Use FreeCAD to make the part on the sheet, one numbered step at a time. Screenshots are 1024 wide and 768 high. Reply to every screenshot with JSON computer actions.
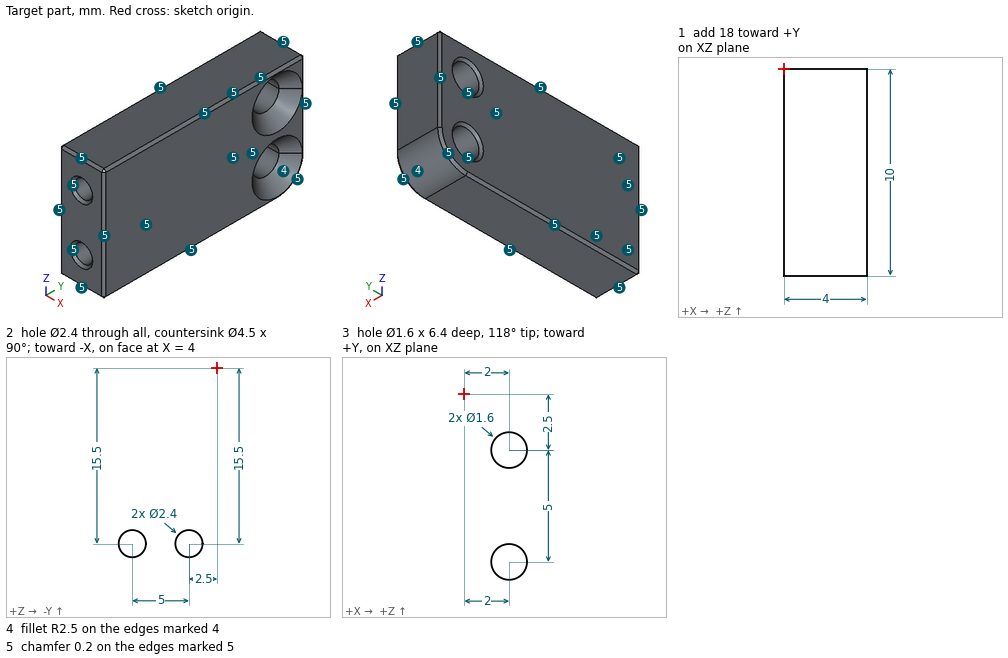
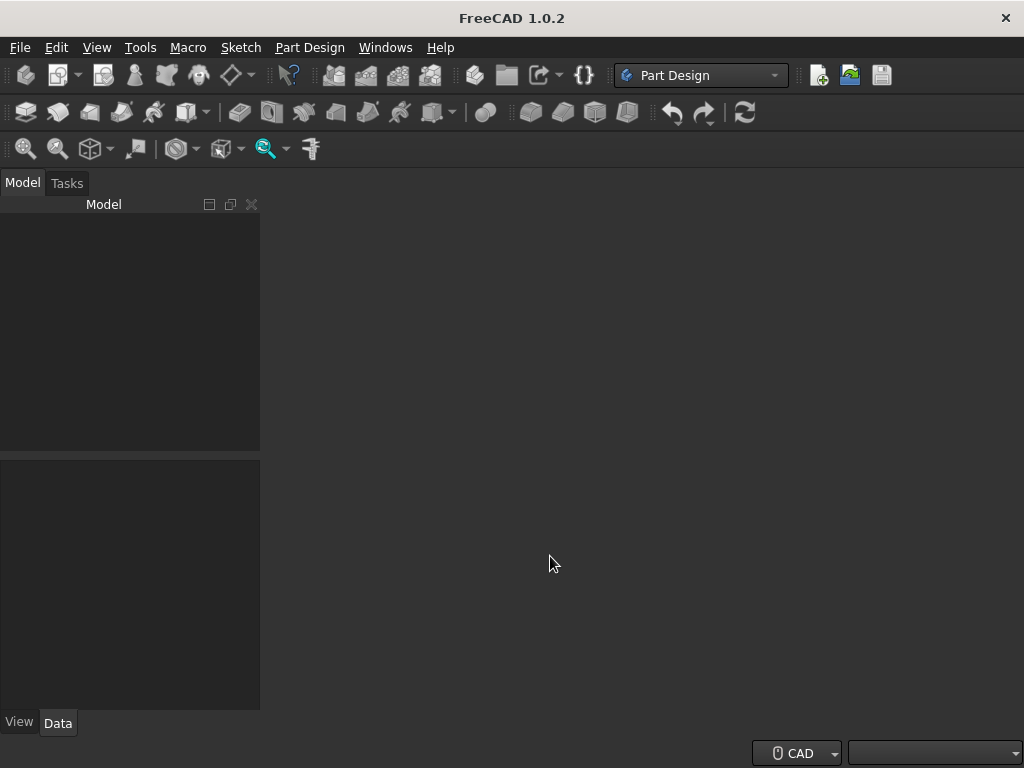
{"action": "left_click", "coordinate": [818, 76]}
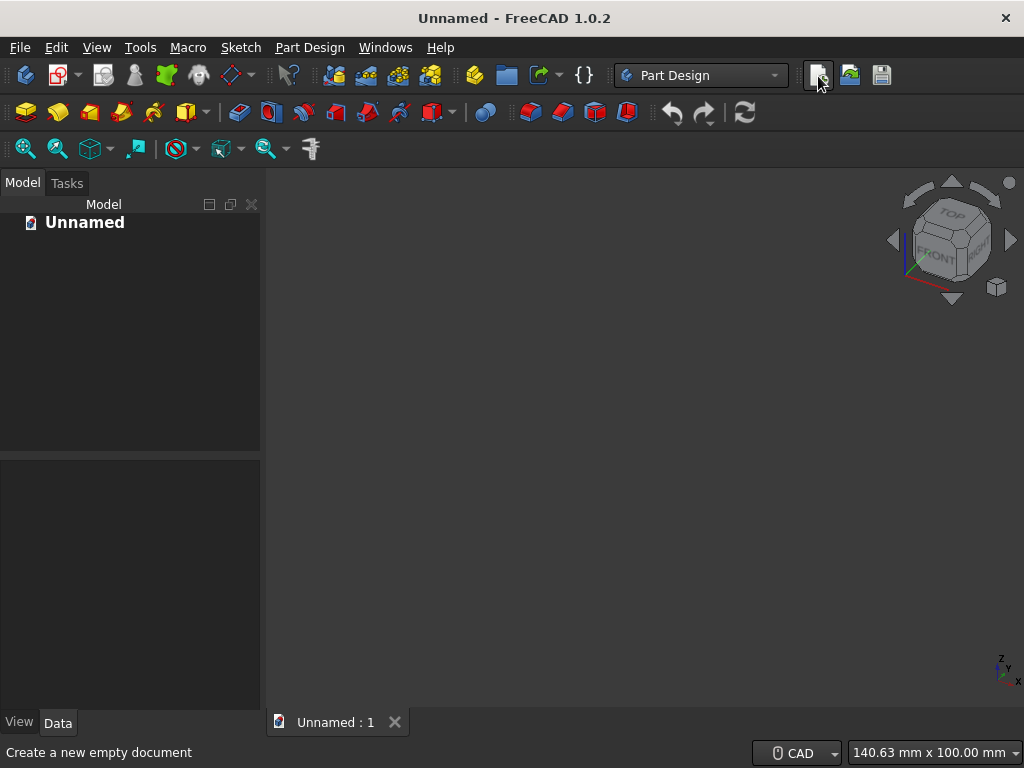
{"action": "left_click", "coordinate": [58, 76]}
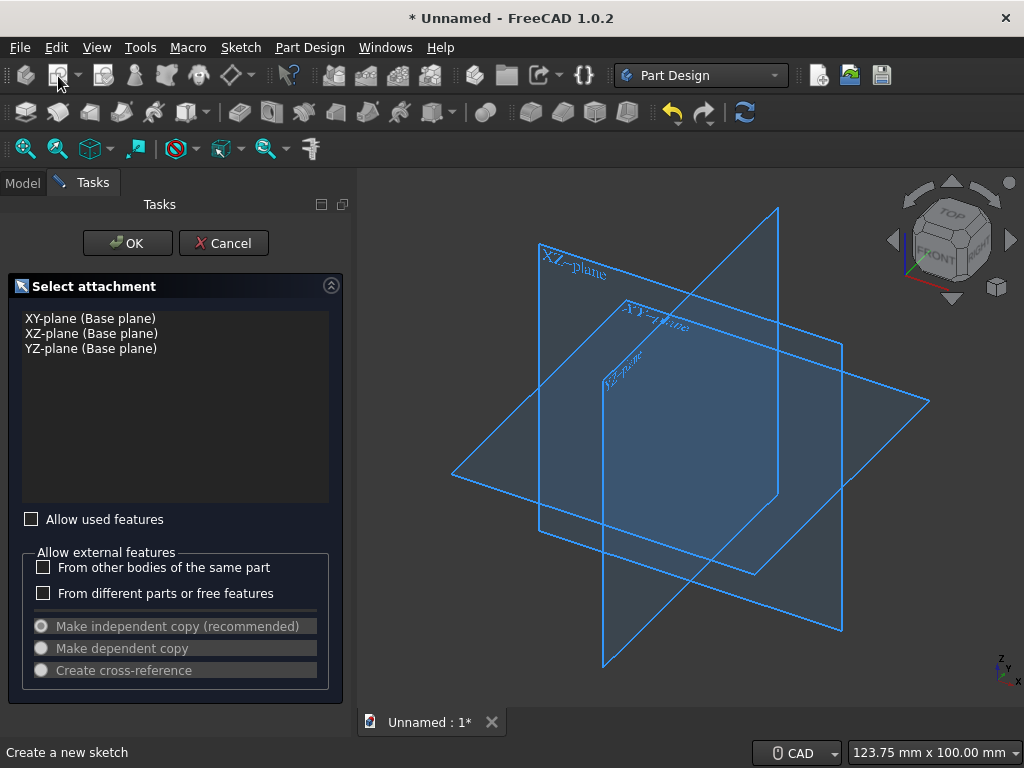
{"action": "left_click", "coordinate": [82, 334]}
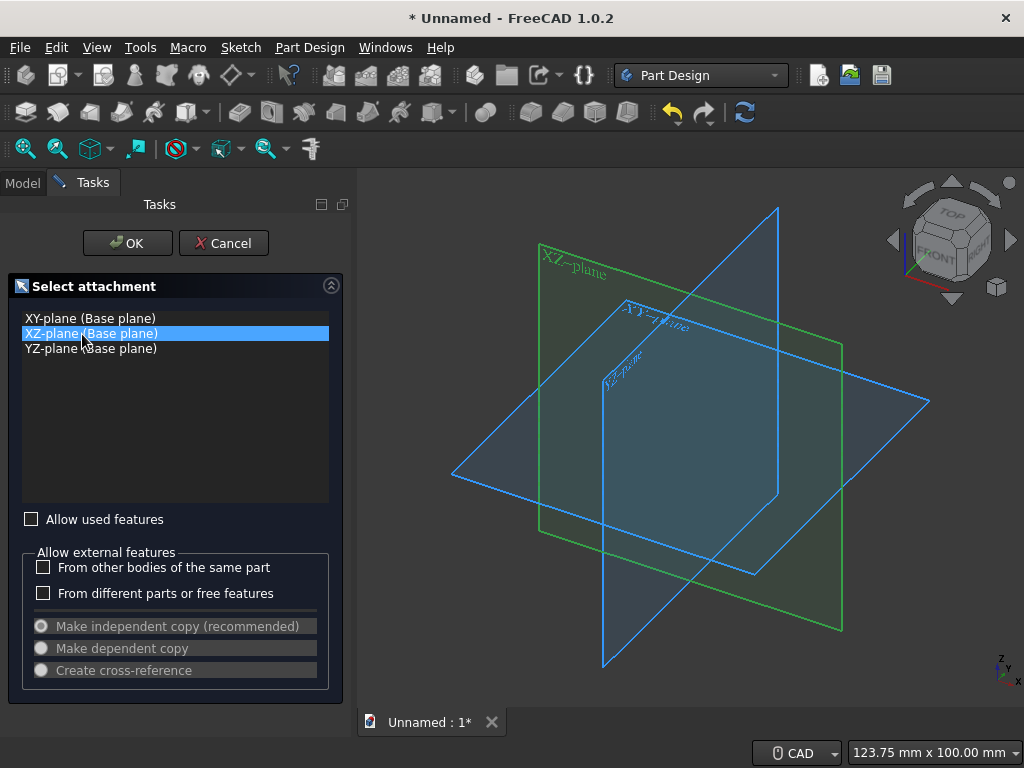
{"action": "left_click", "coordinate": [128, 243]}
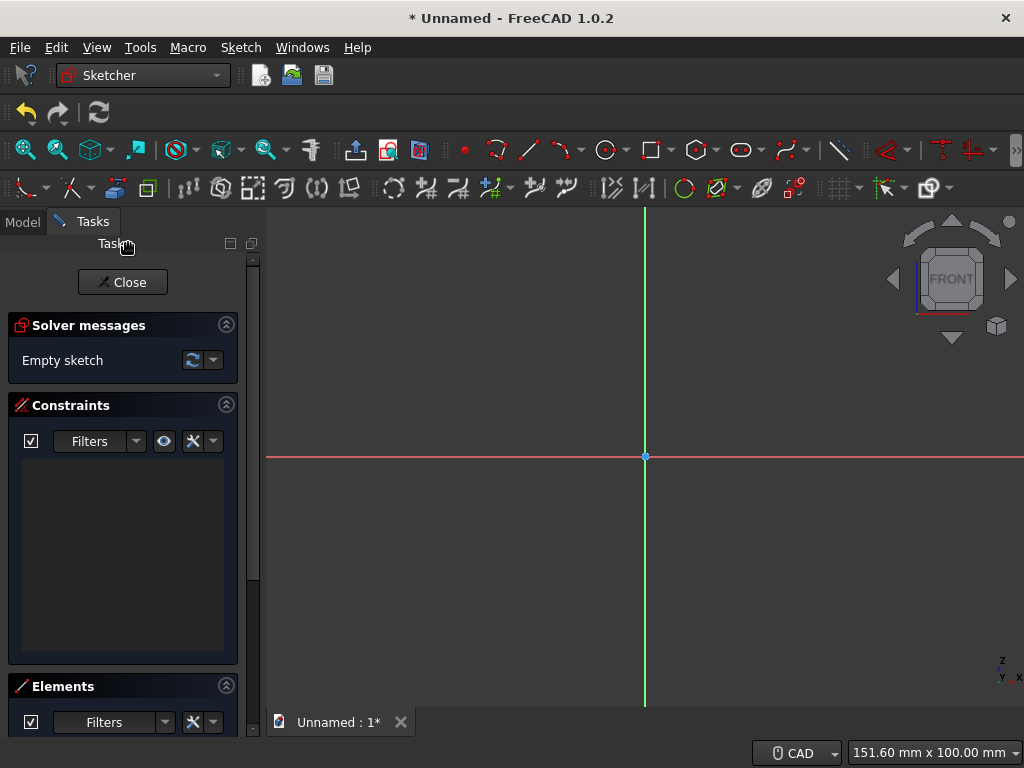
{"action": "scroll", "coordinate": [671, 487], "scroll_direction": "up", "scroll_amount": 9}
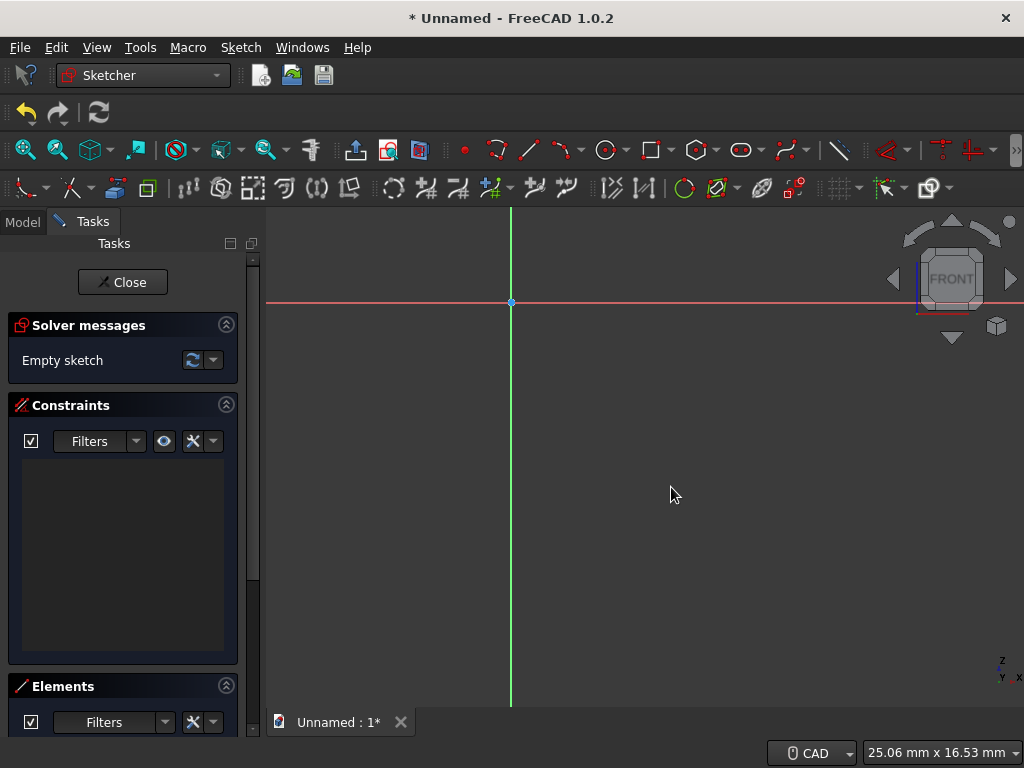
{"action": "left_click", "coordinate": [652, 150]}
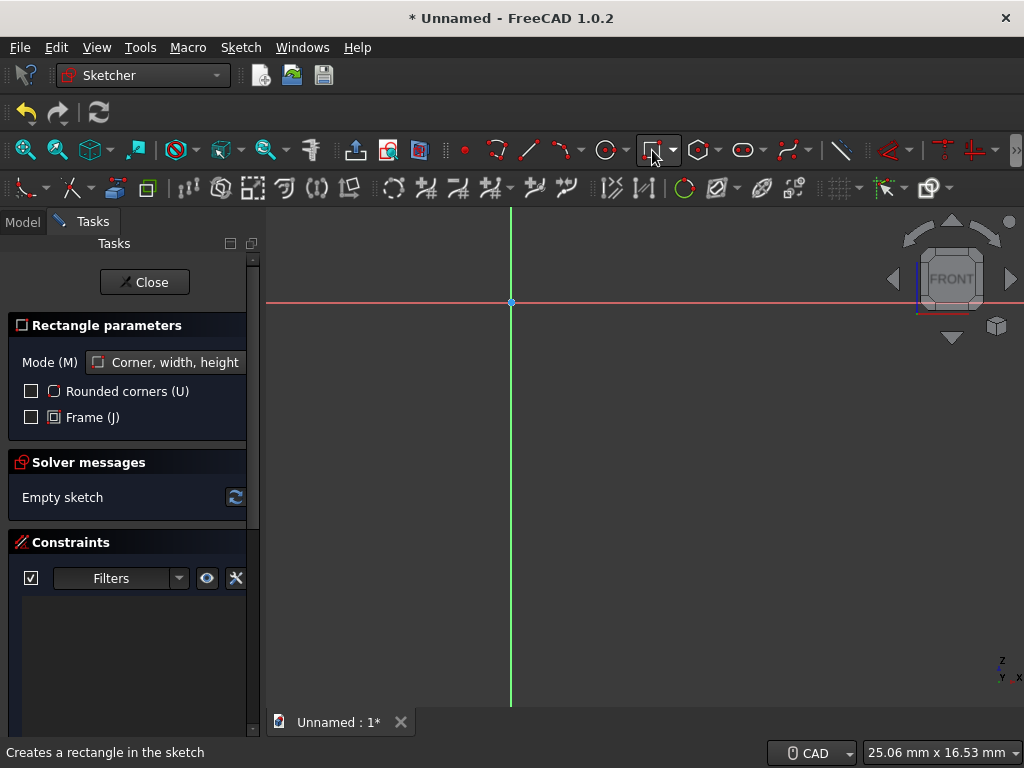
{"action": "left_click", "coordinate": [511, 303]}
{"action": "mouse_move", "coordinate": [632, 605]}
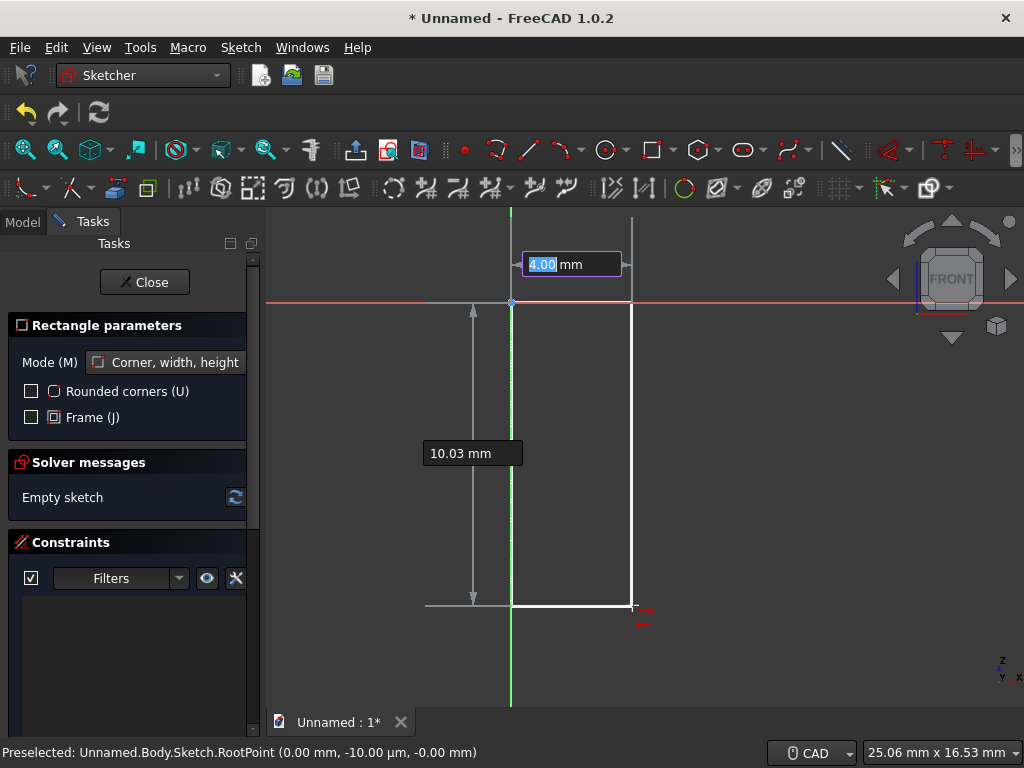
{"action": "type", "text": "4"}
{"action": "key", "text": "Tab"}
{"action": "type", "text": "10"}
{"action": "key", "text": "Return"}
{"action": "key", "text": "Escape"}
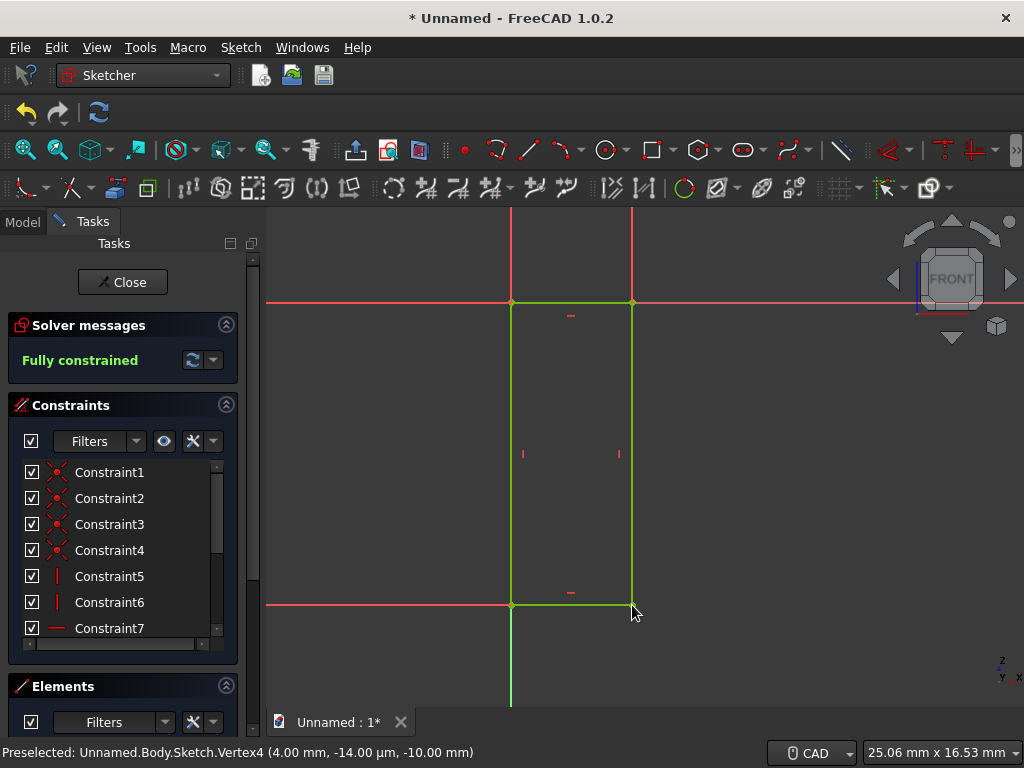
{"action": "left_click", "coordinate": [123, 282]}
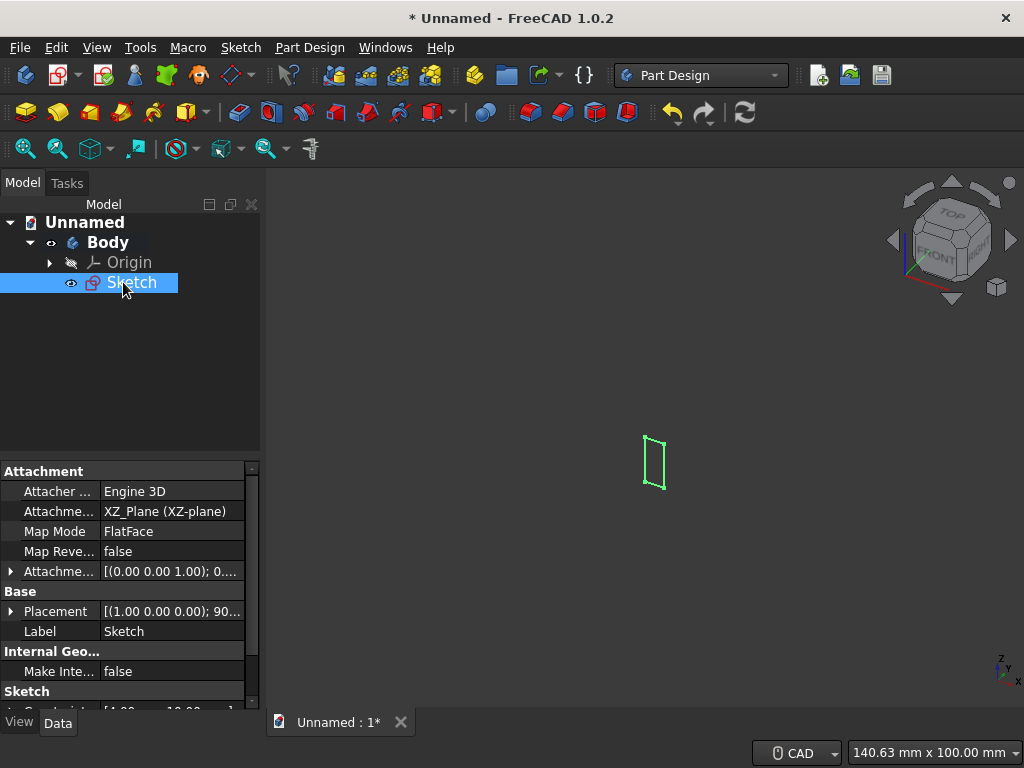
{"action": "left_click", "coordinate": [26, 112]}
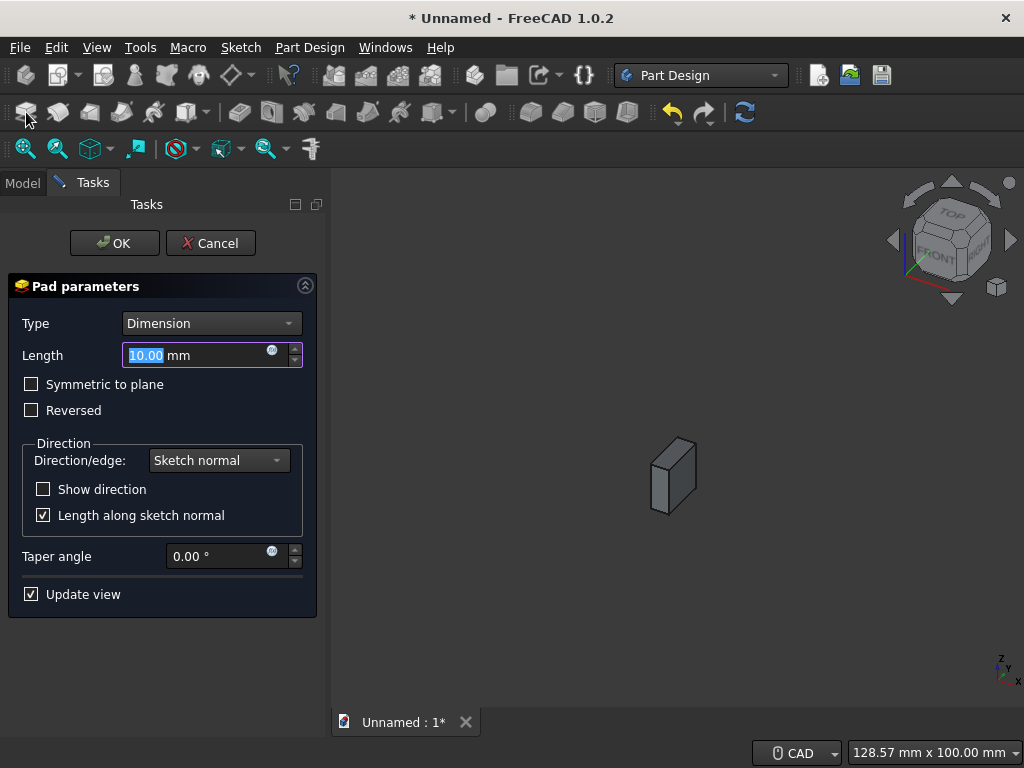
{"action": "type", "text": "18"}
{"action": "key", "text": "Tab"}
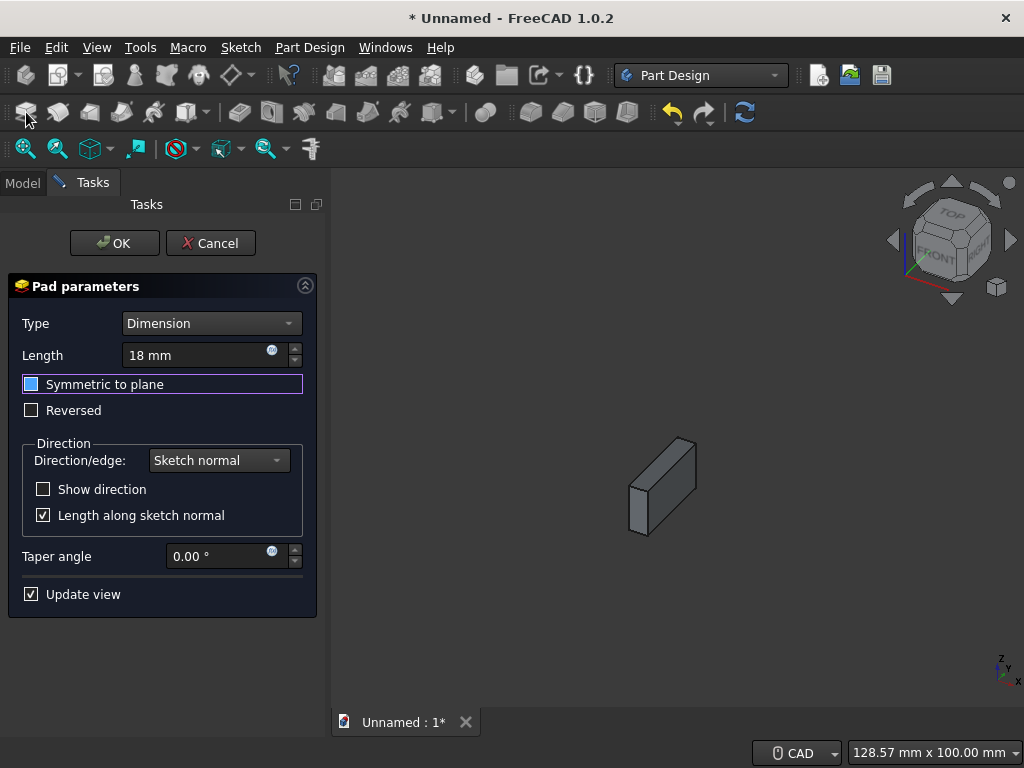
{"action": "left_click", "coordinate": [30, 410]}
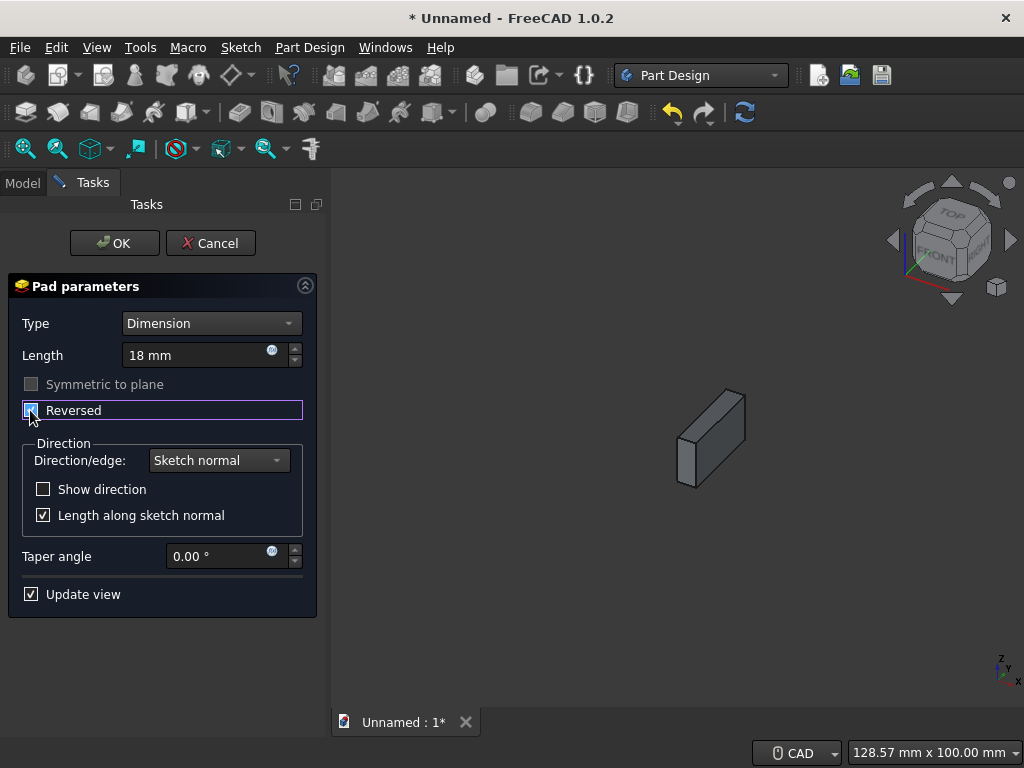
{"action": "left_click", "coordinate": [115, 243]}